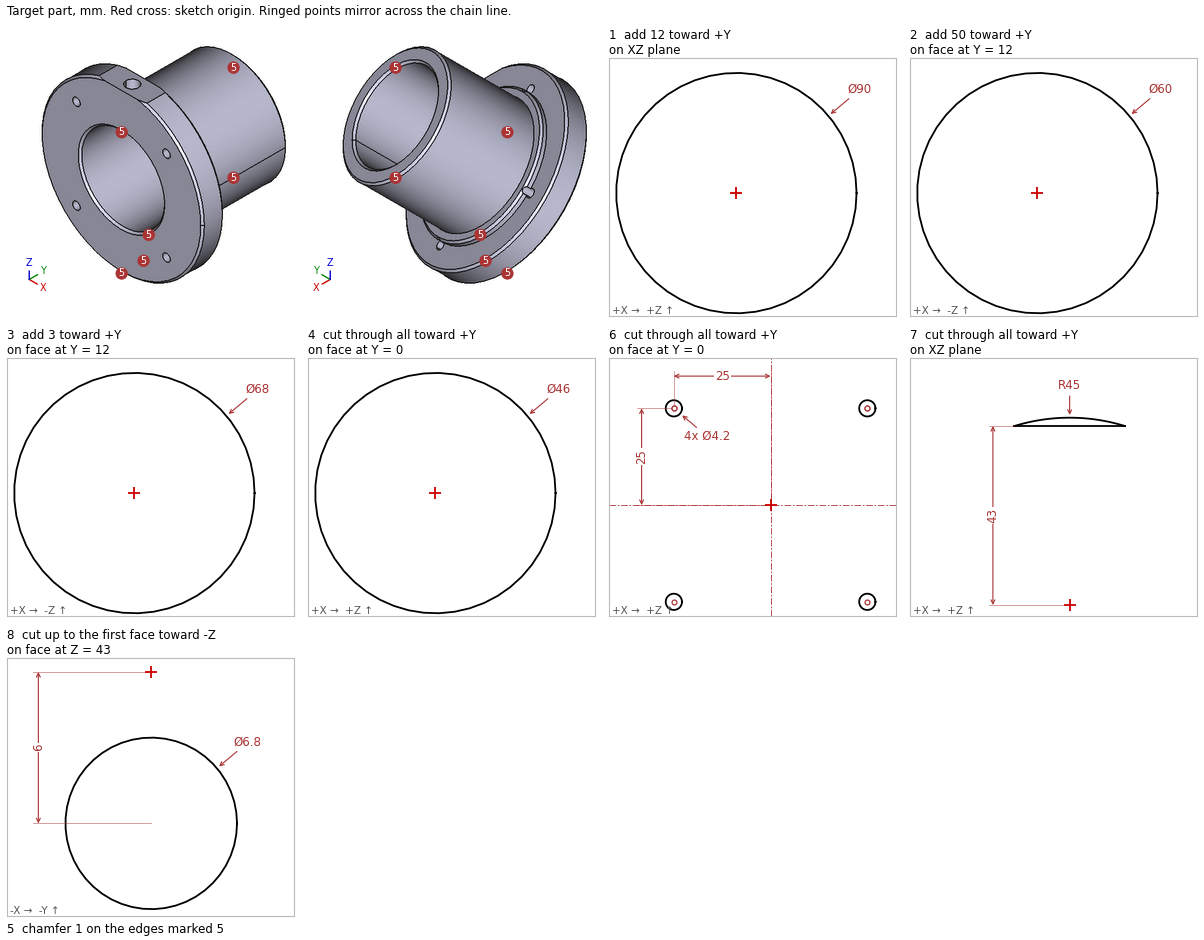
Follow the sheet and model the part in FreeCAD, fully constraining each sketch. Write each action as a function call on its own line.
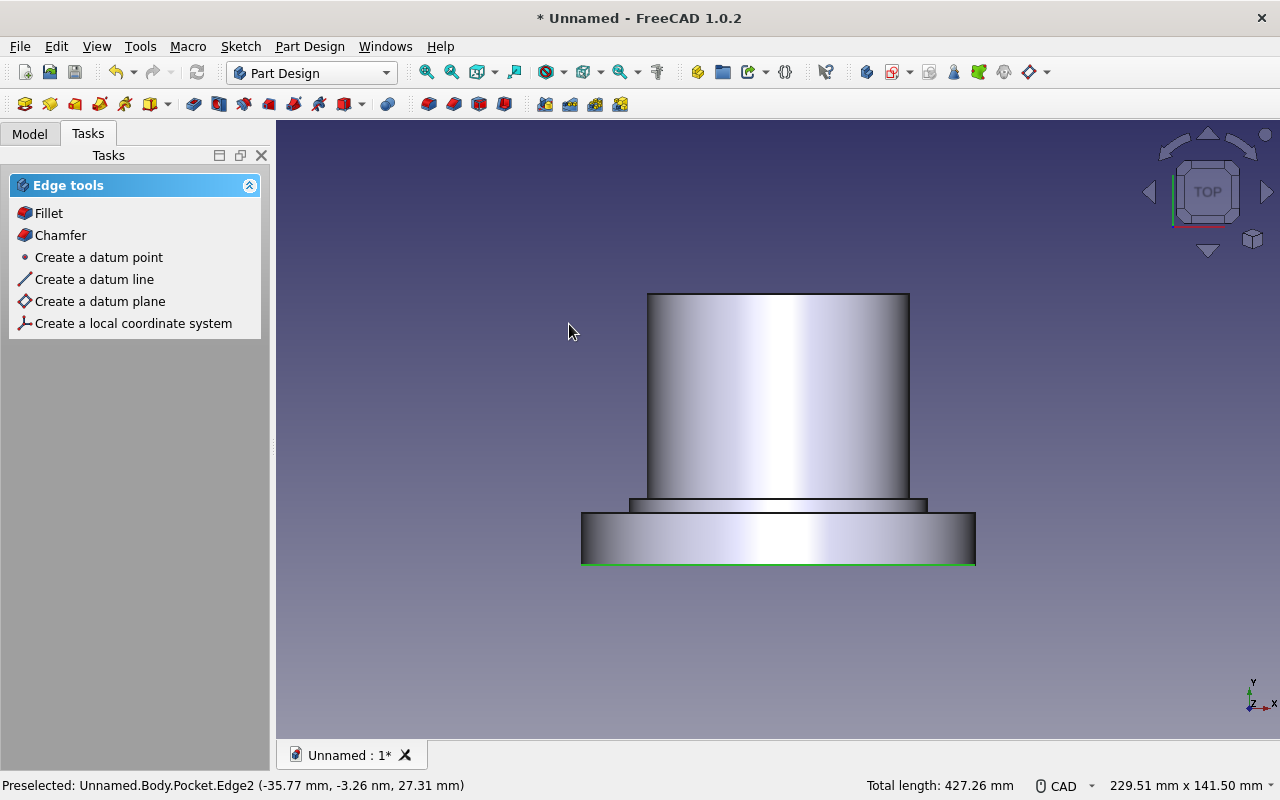
click(427, 72)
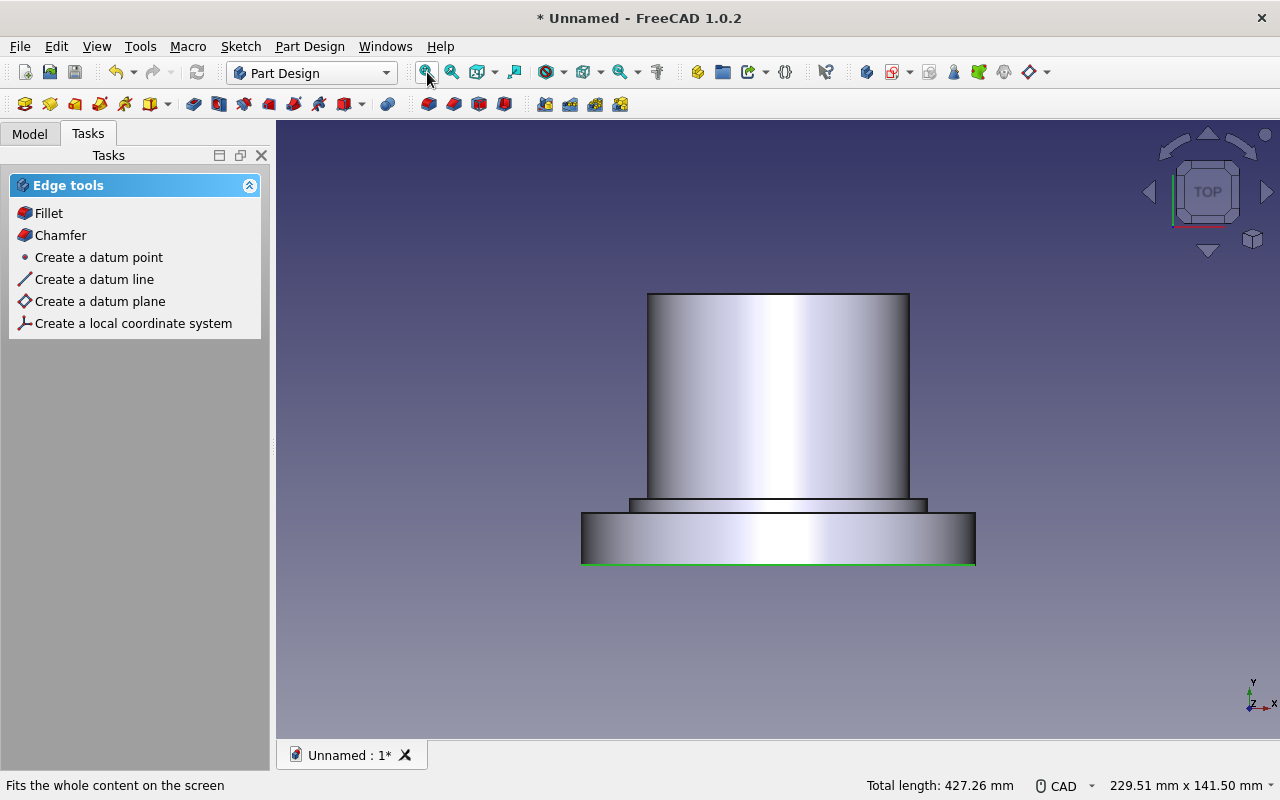
click(657, 498, ctrl)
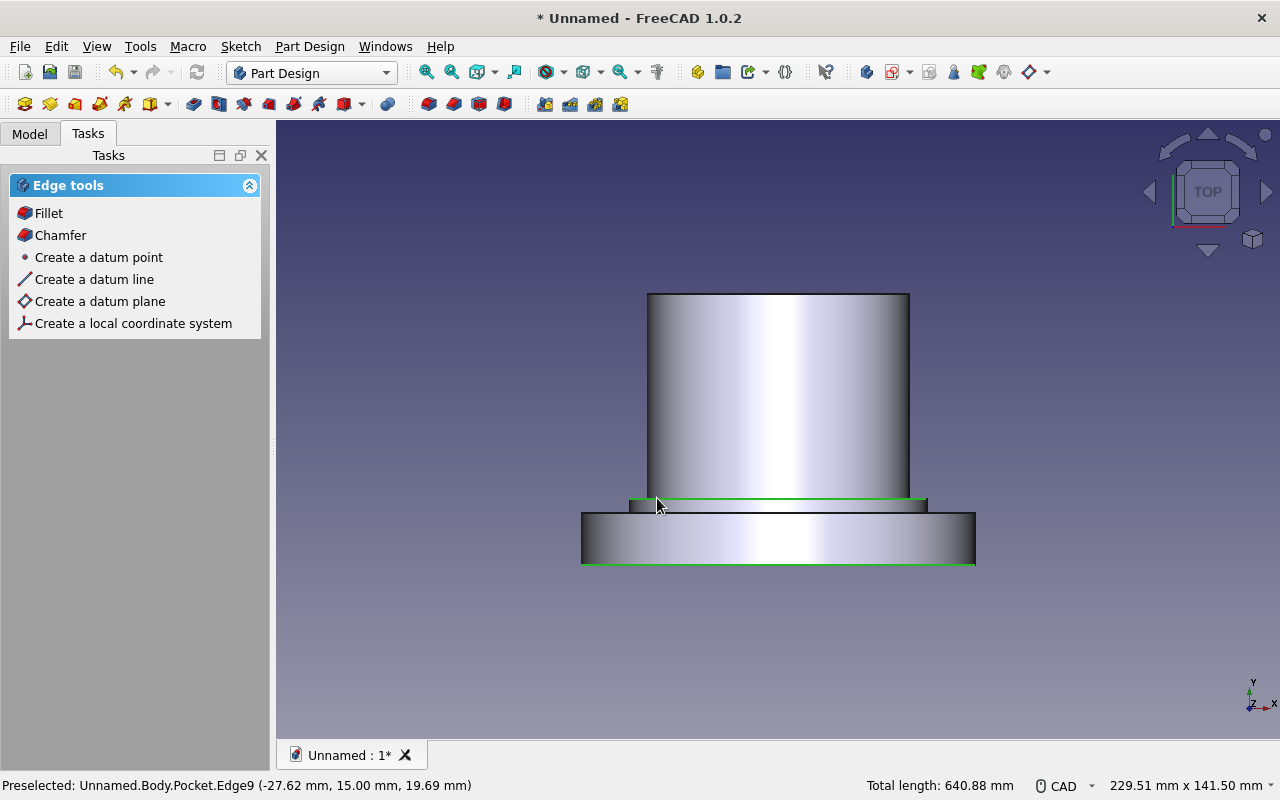
click(619, 512, ctrl)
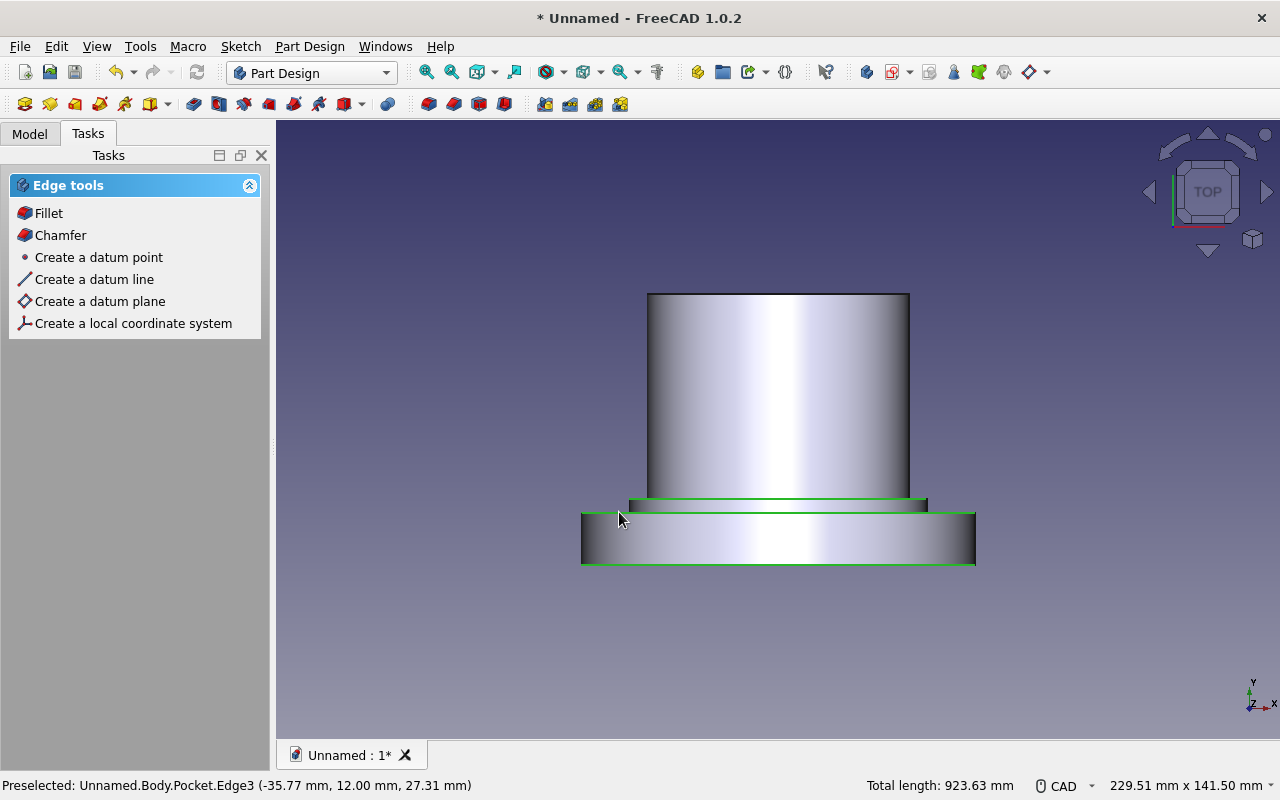
click(672, 293, ctrl)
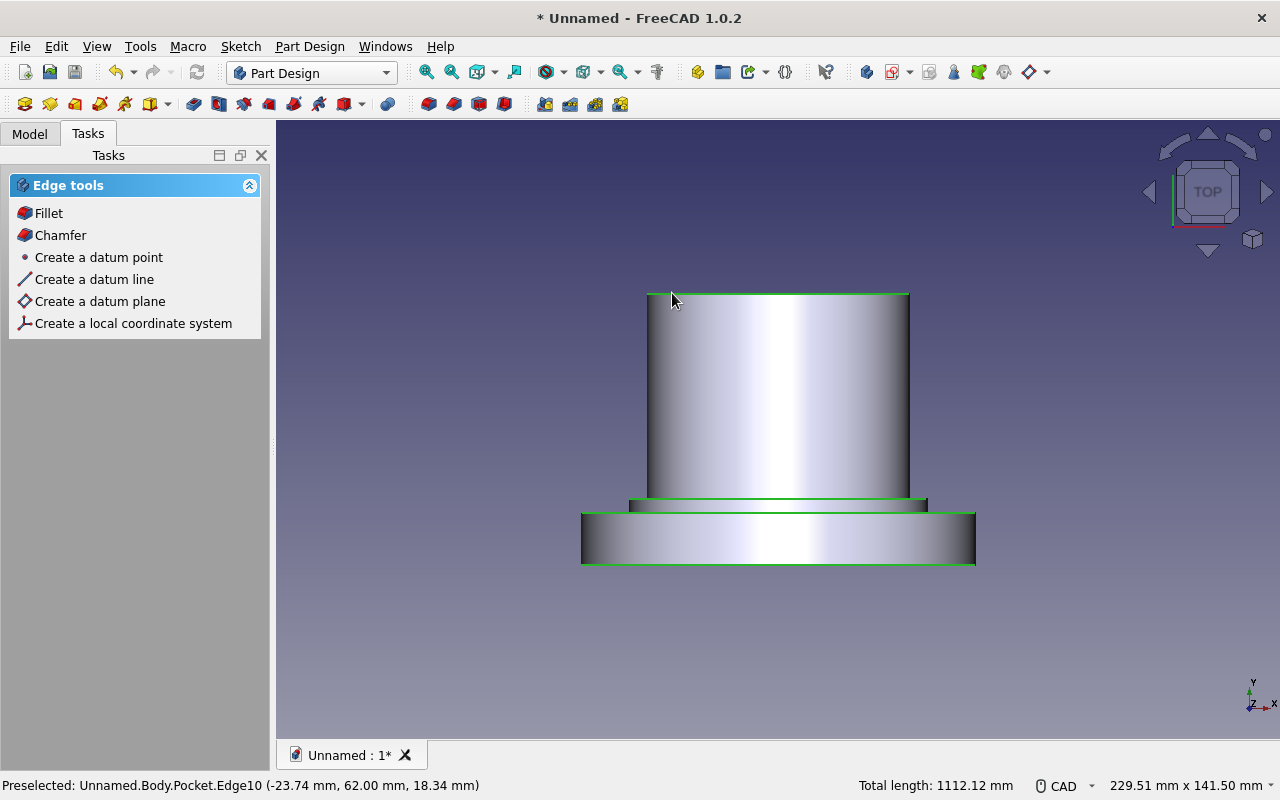
key(0)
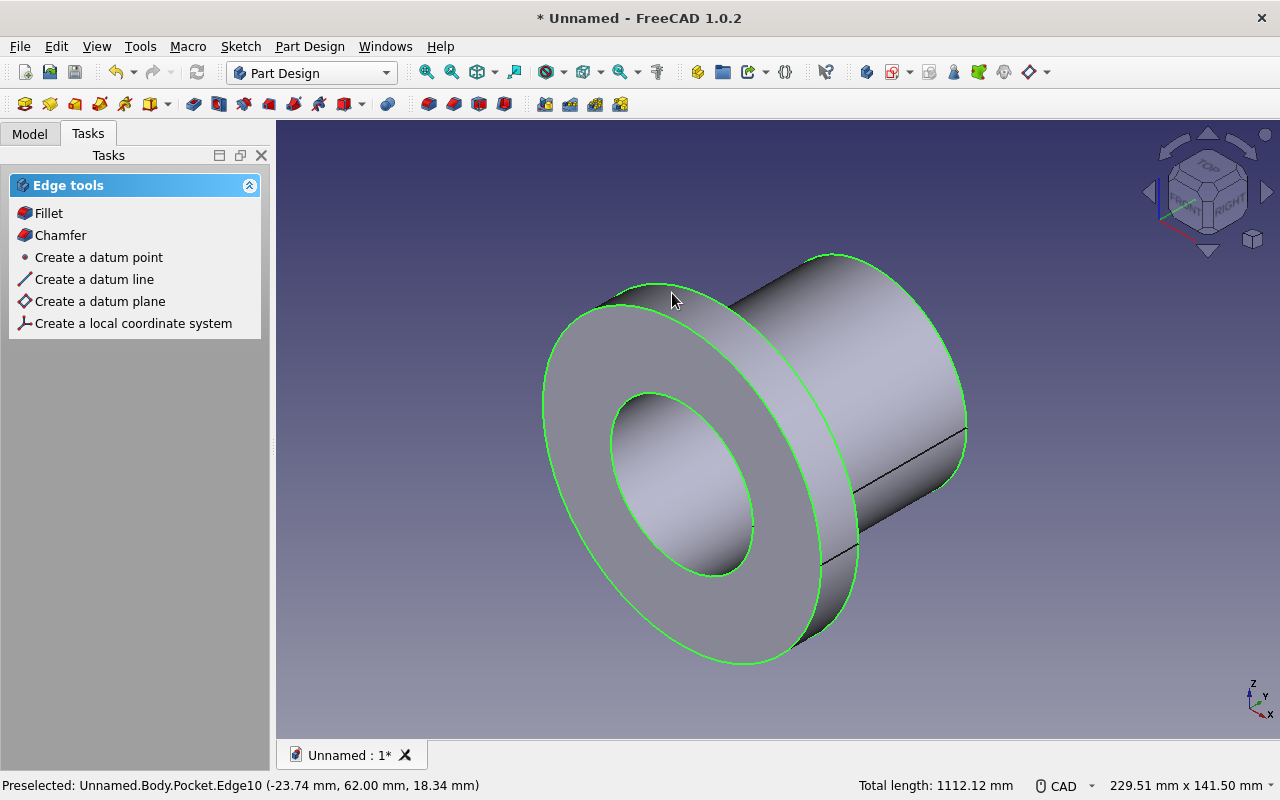
key(1)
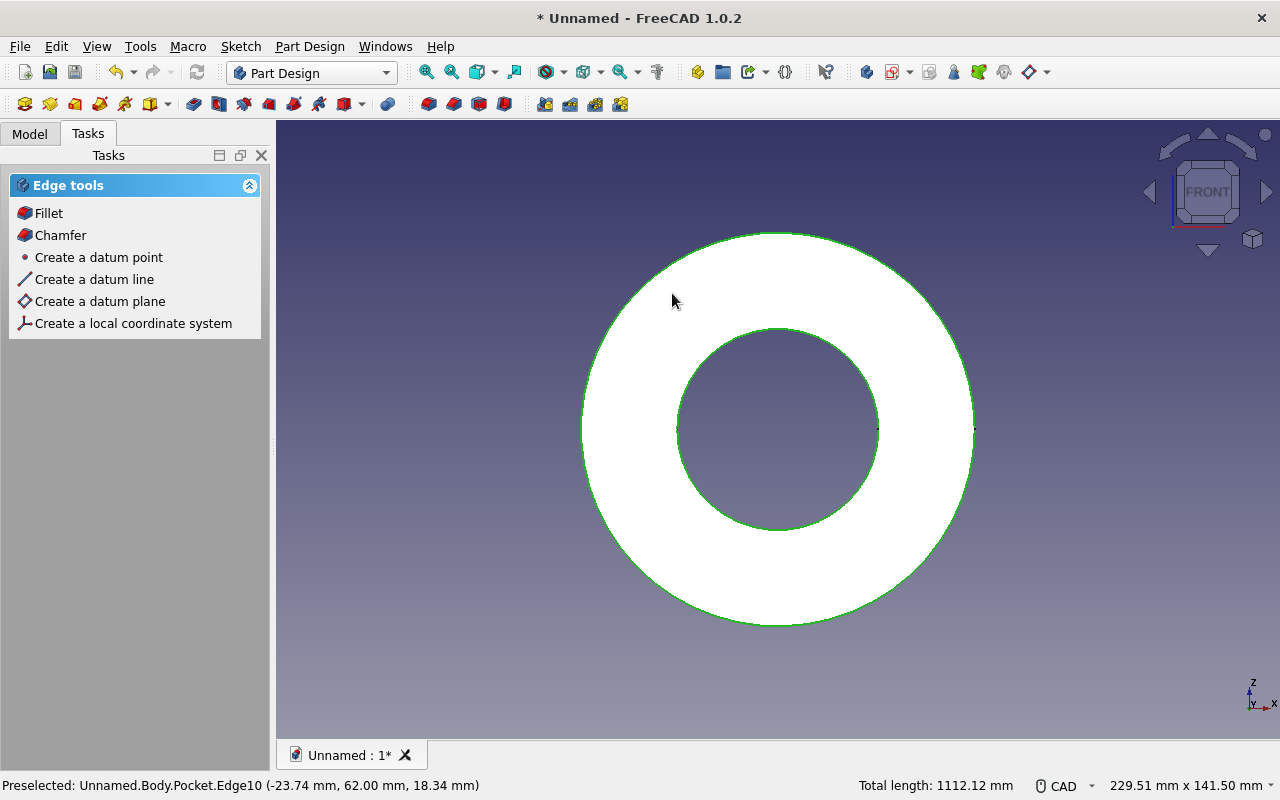
key(3)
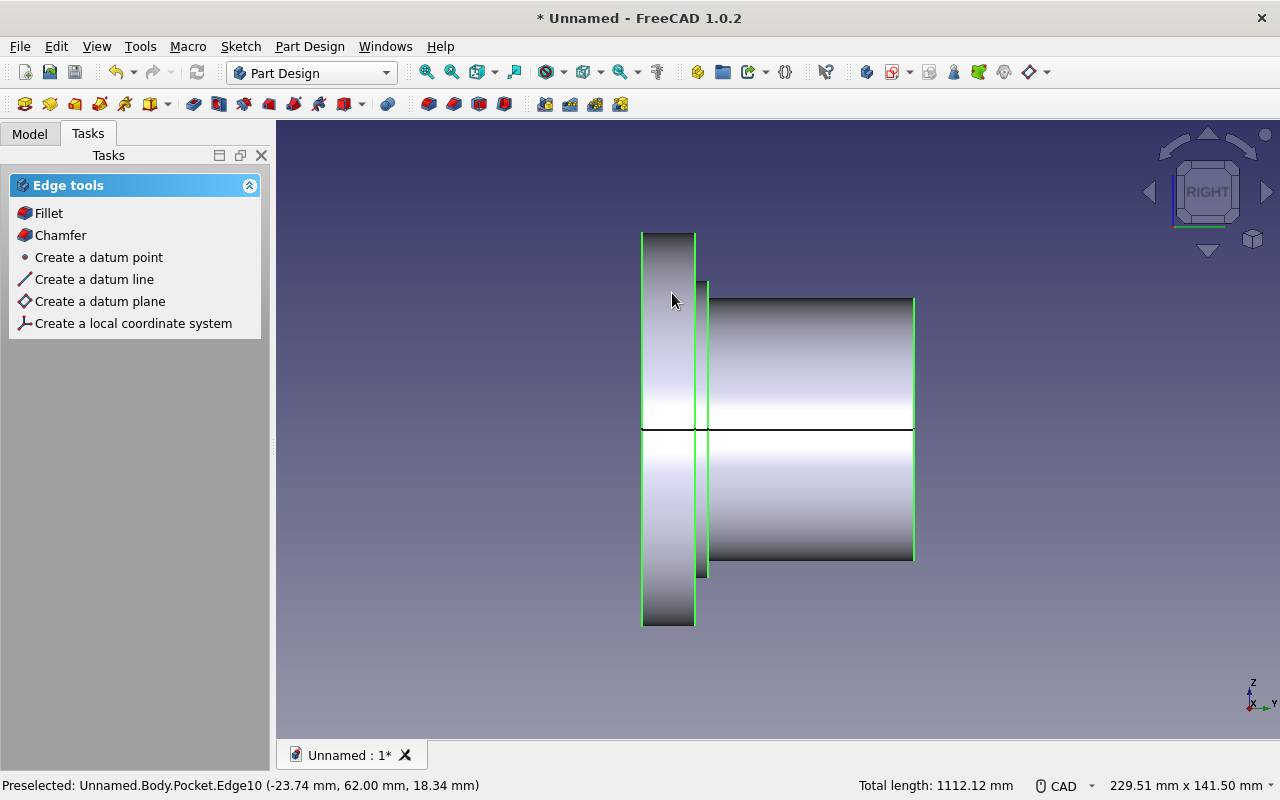
key(5)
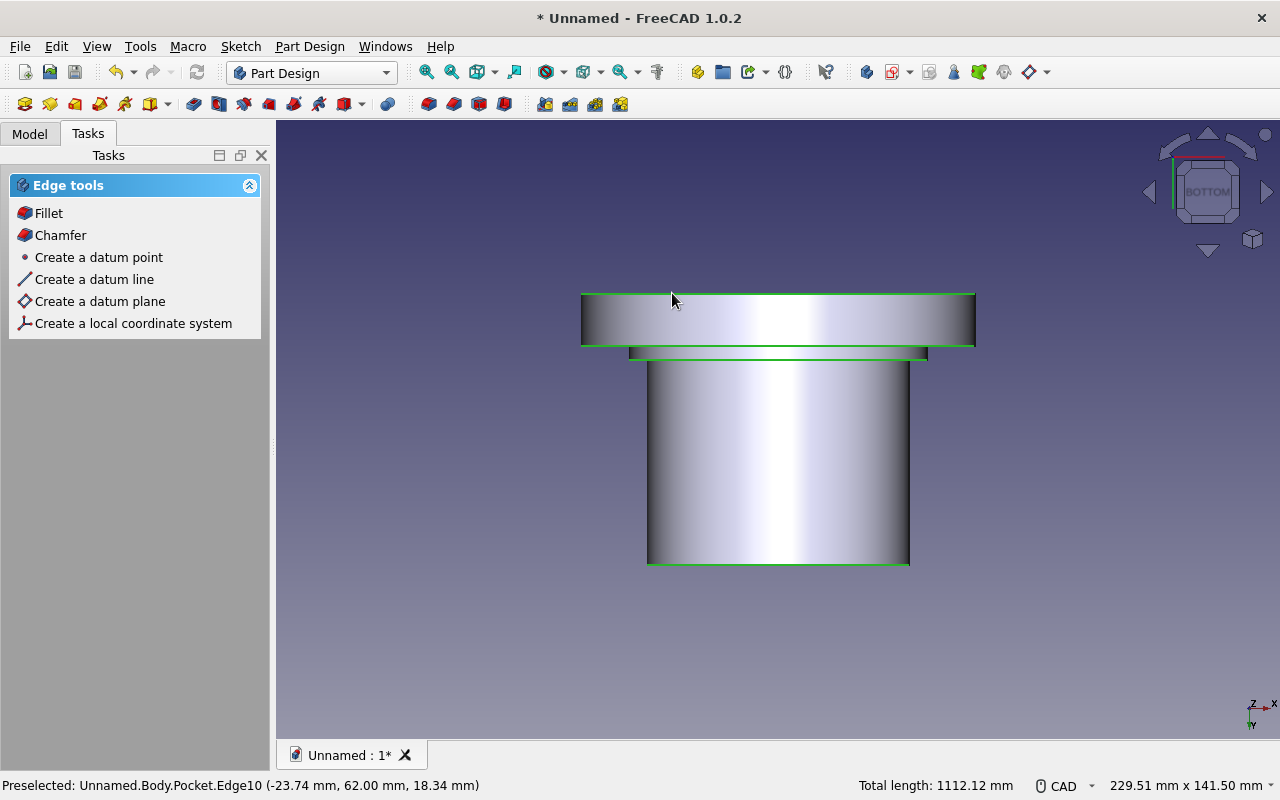
click(427, 72)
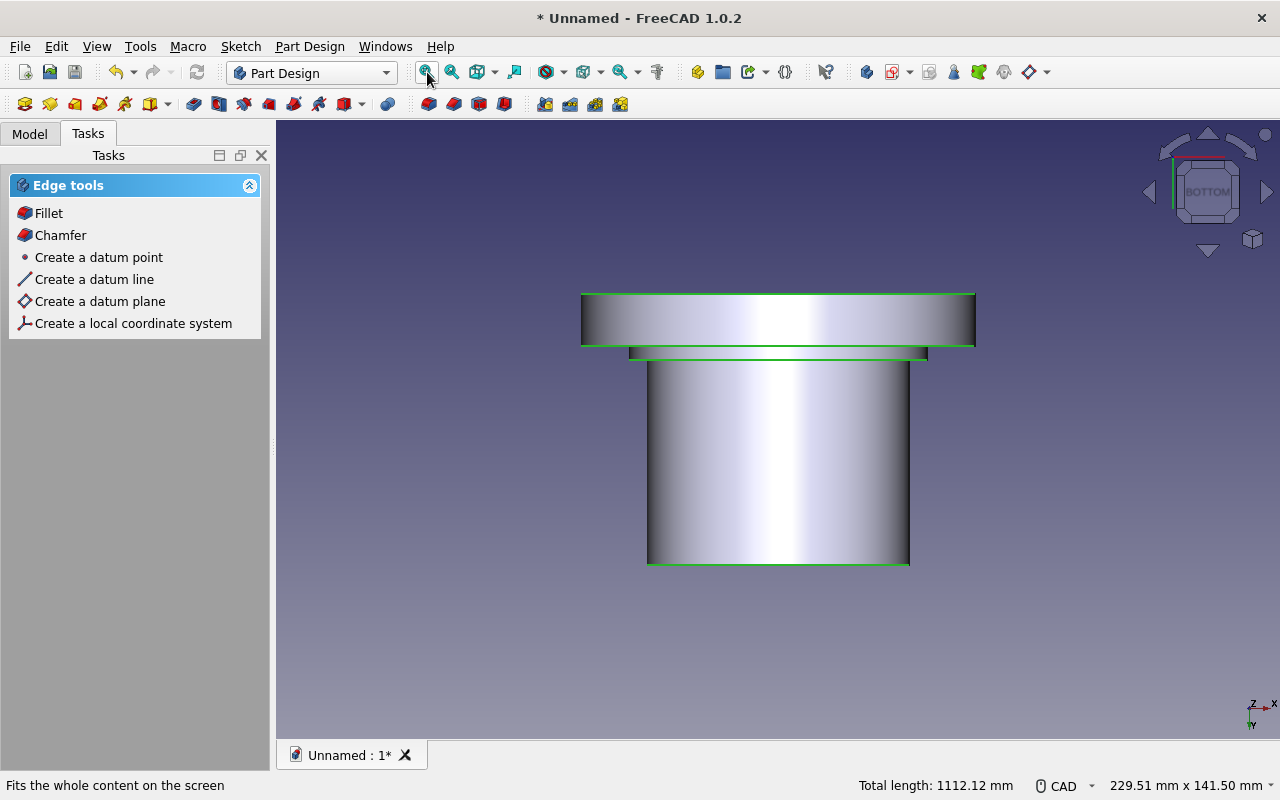
key(4)